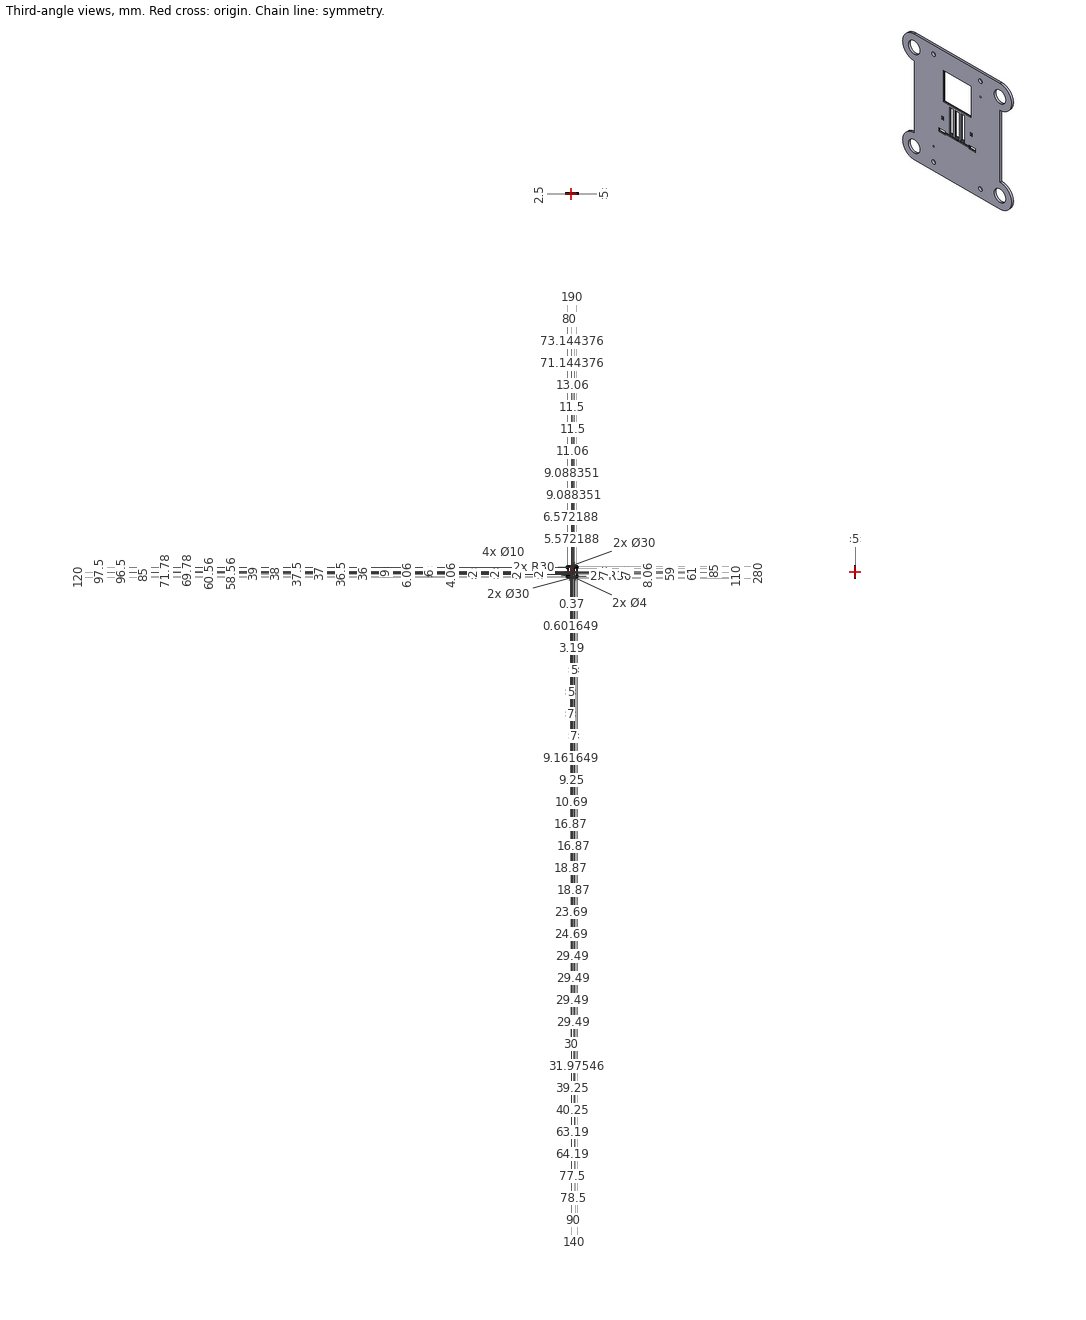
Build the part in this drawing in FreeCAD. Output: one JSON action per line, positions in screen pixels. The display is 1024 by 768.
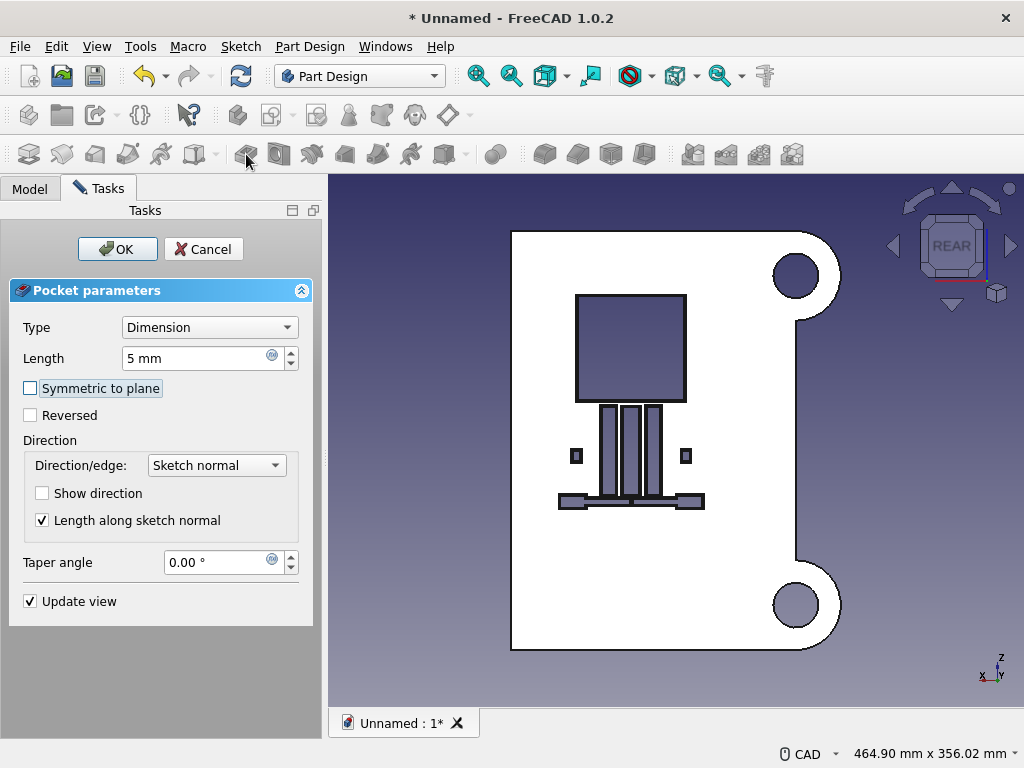
{"action": "left_click", "coordinate": [118, 249]}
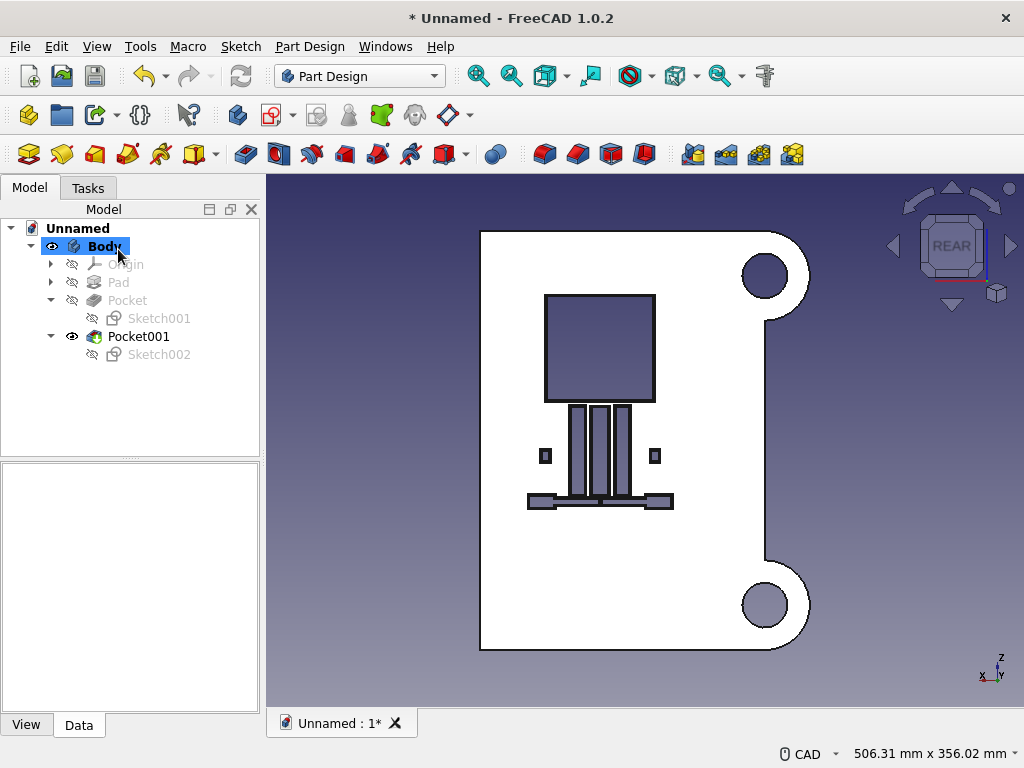
{"action": "left_click", "coordinate": [692, 559]}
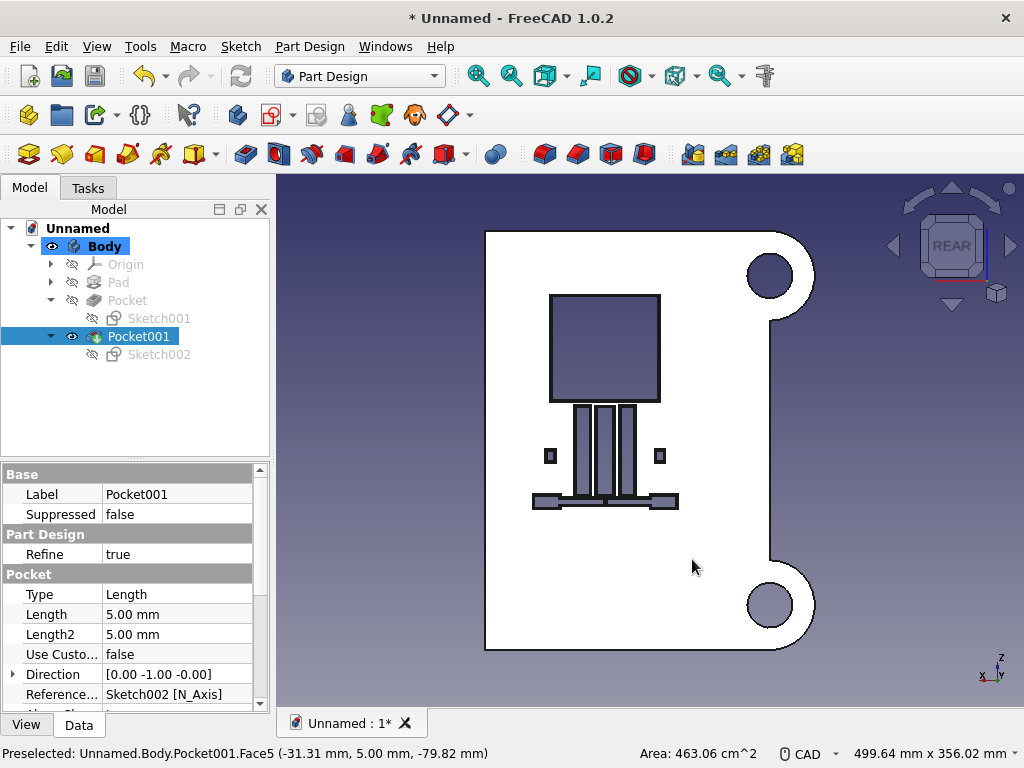
{"action": "left_click", "coordinate": [270, 116]}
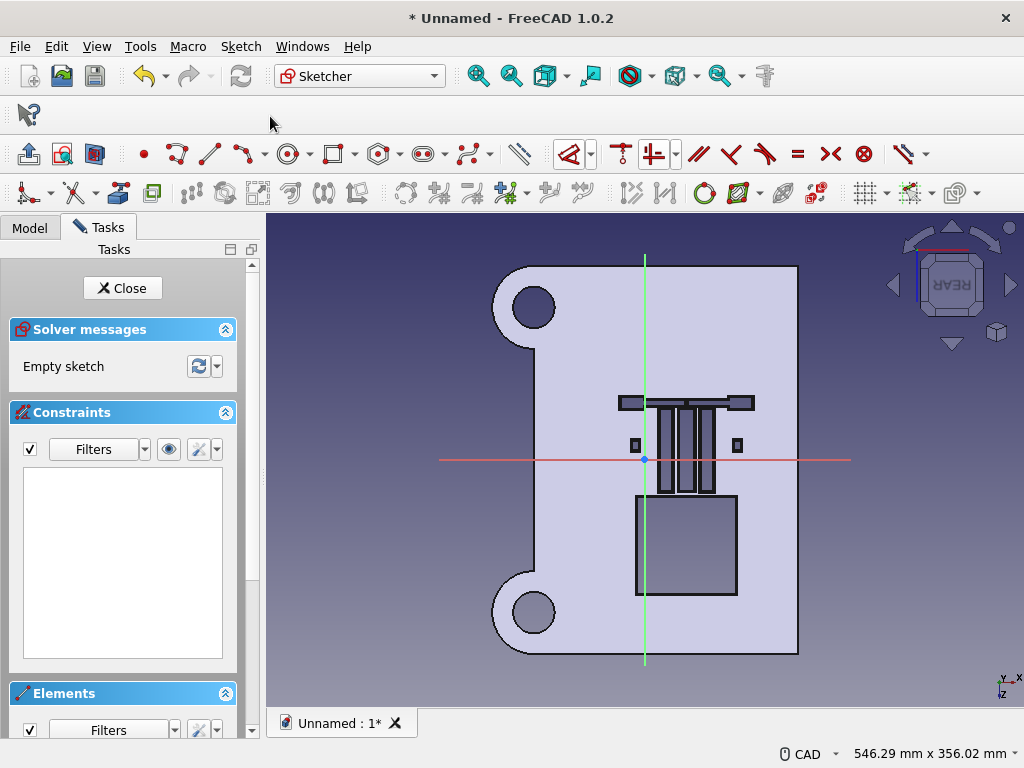
{"action": "key", "text": "g c"}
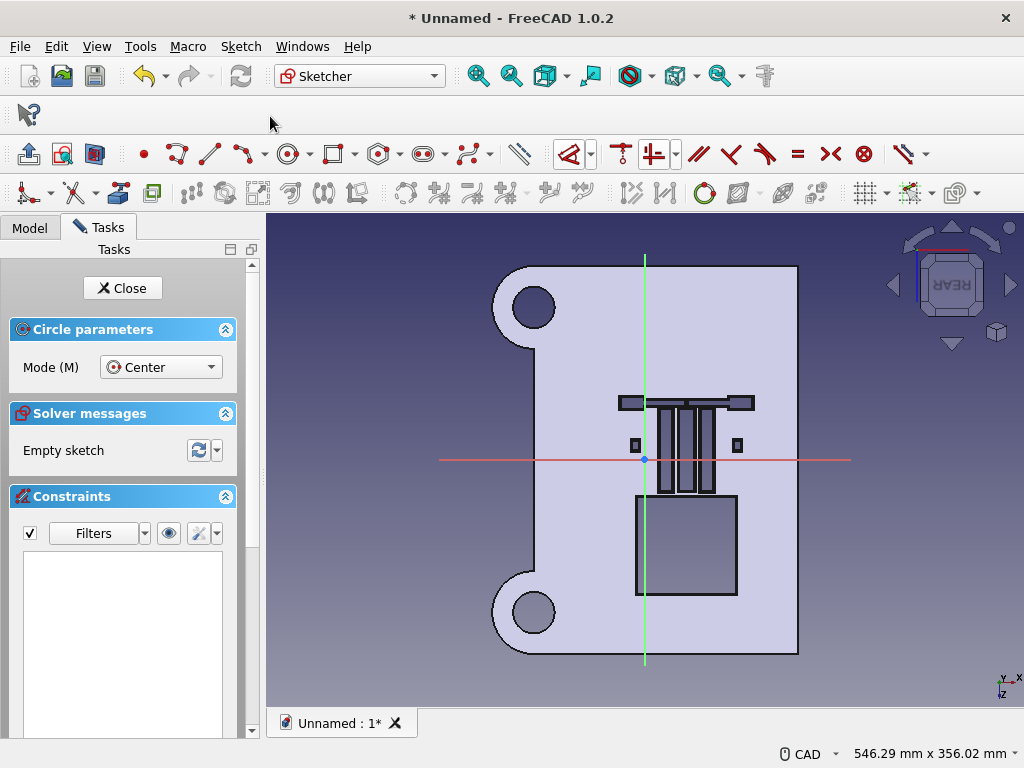
{"action": "scroll", "coordinate": [603, 293], "scroll_direction": "up", "scroll_amount": 6}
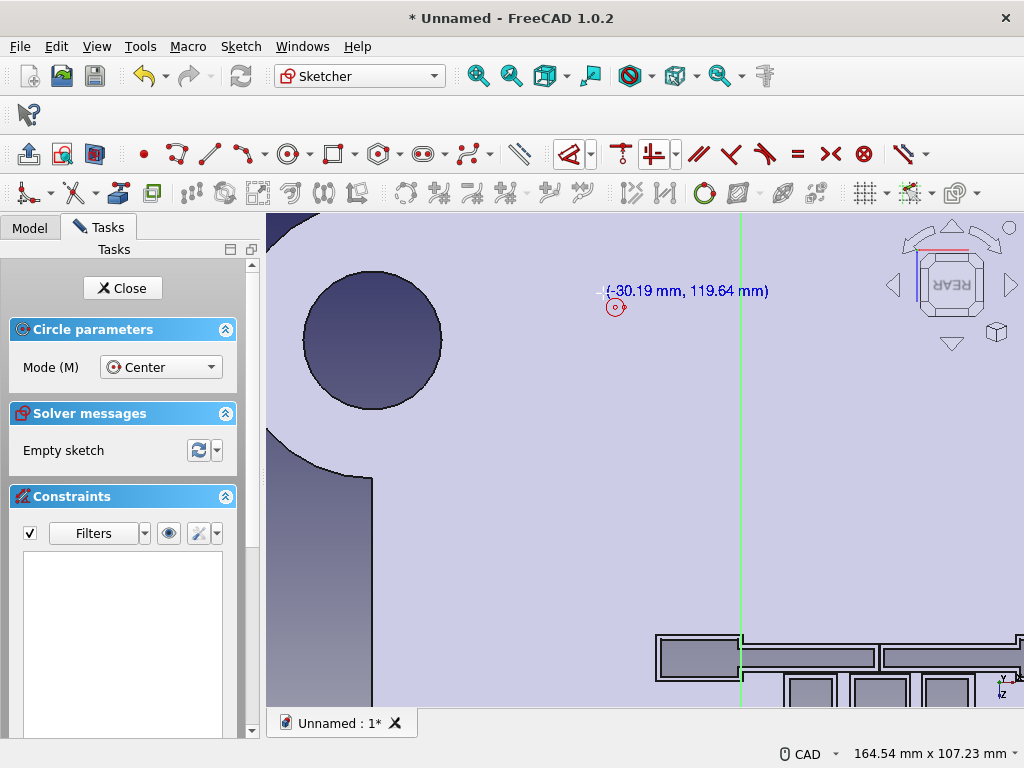
{"action": "left_click", "coordinate": [603, 294]}
{"action": "left_click", "coordinate": [619, 278]}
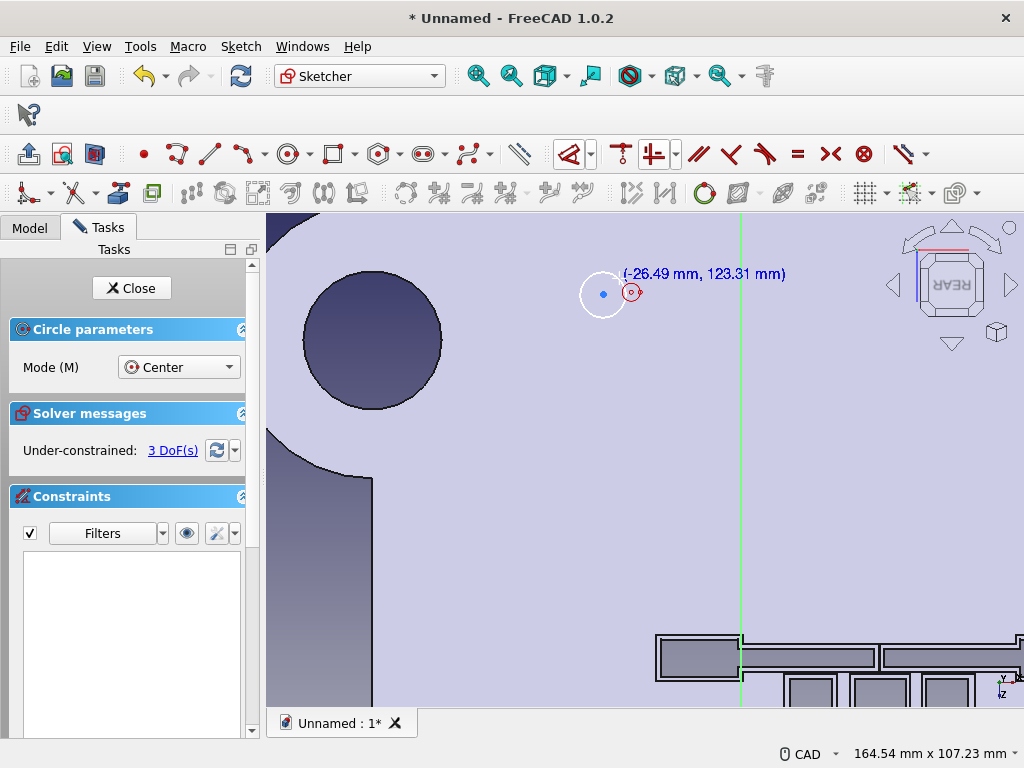
{"action": "scroll", "coordinate": [477, 333], "scroll_direction": "down", "scroll_amount": 7}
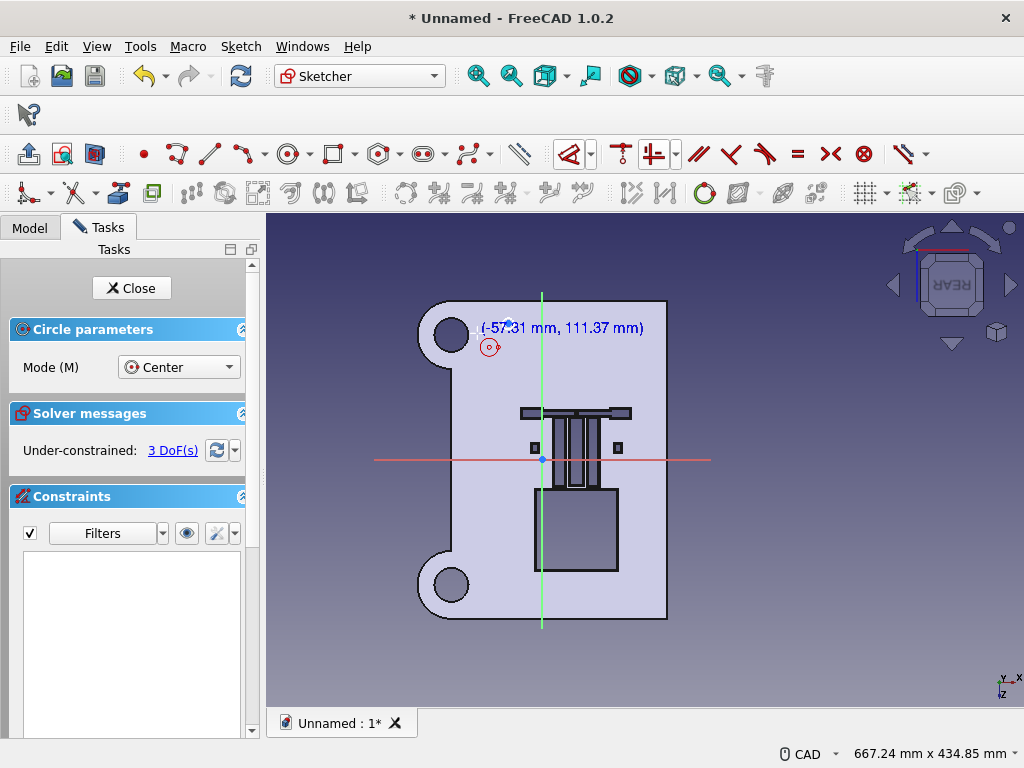
{"action": "scroll", "coordinate": [645, 324], "scroll_direction": "up", "scroll_amount": 7}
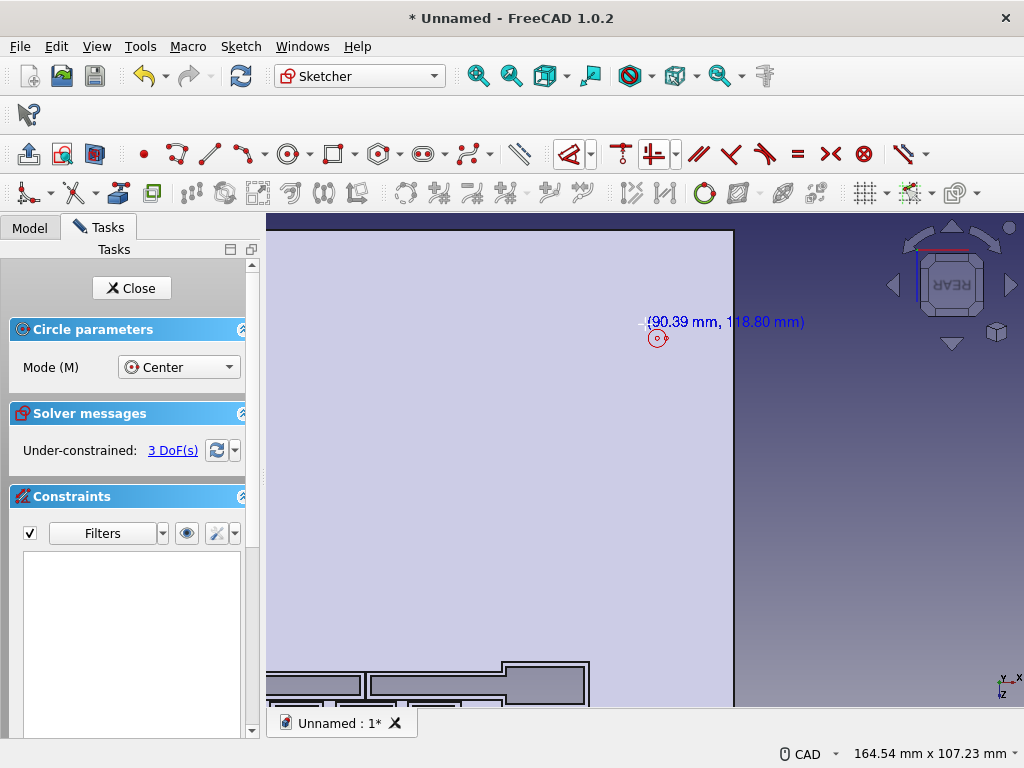
{"action": "left_click", "coordinate": [642, 322]}
{"action": "left_click", "coordinate": [658, 306]}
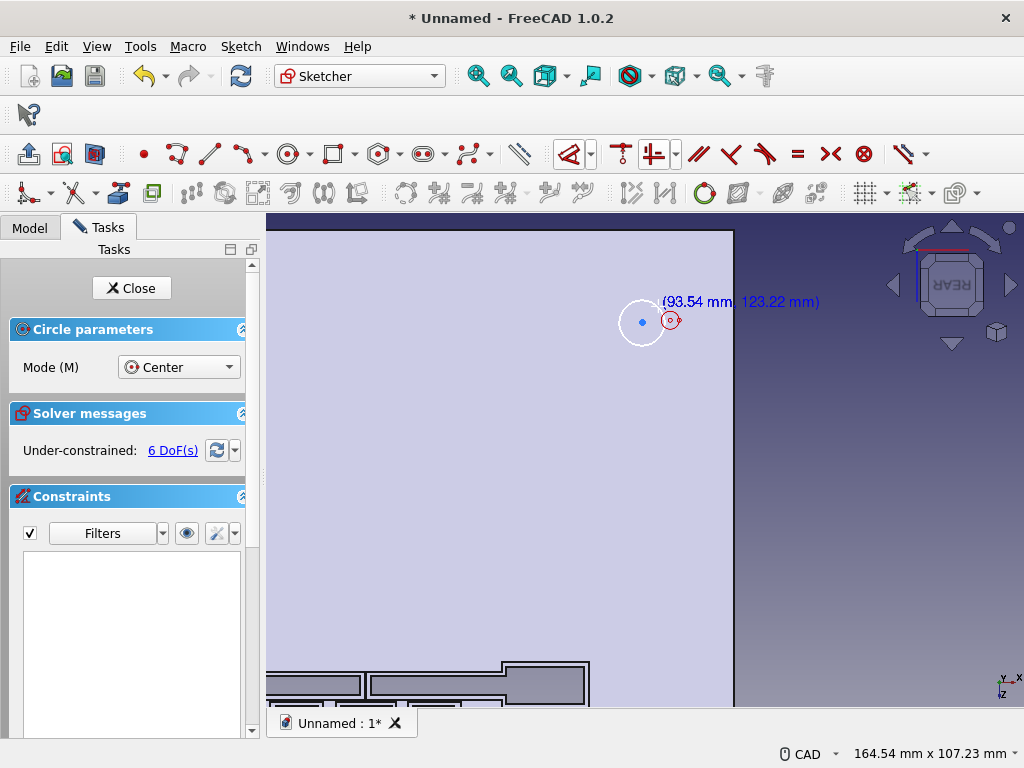
{"action": "scroll", "coordinate": [646, 324], "scroll_direction": "down", "scroll_amount": 7}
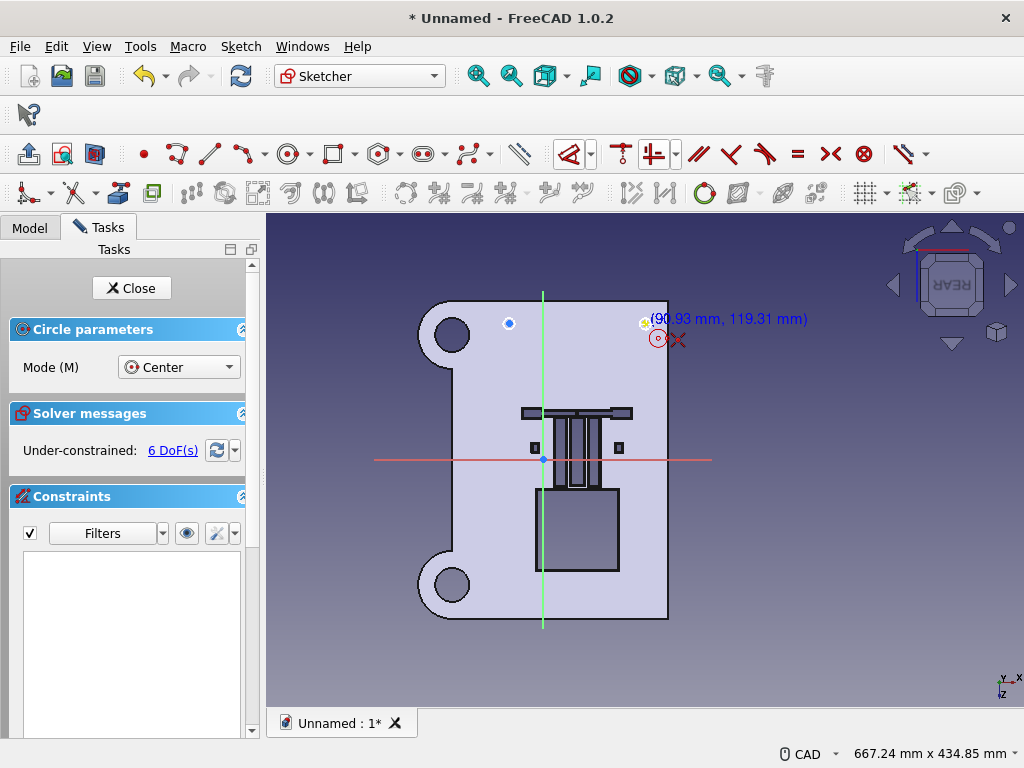
{"action": "scroll", "coordinate": [645, 596], "scroll_direction": "up", "scroll_amount": 7}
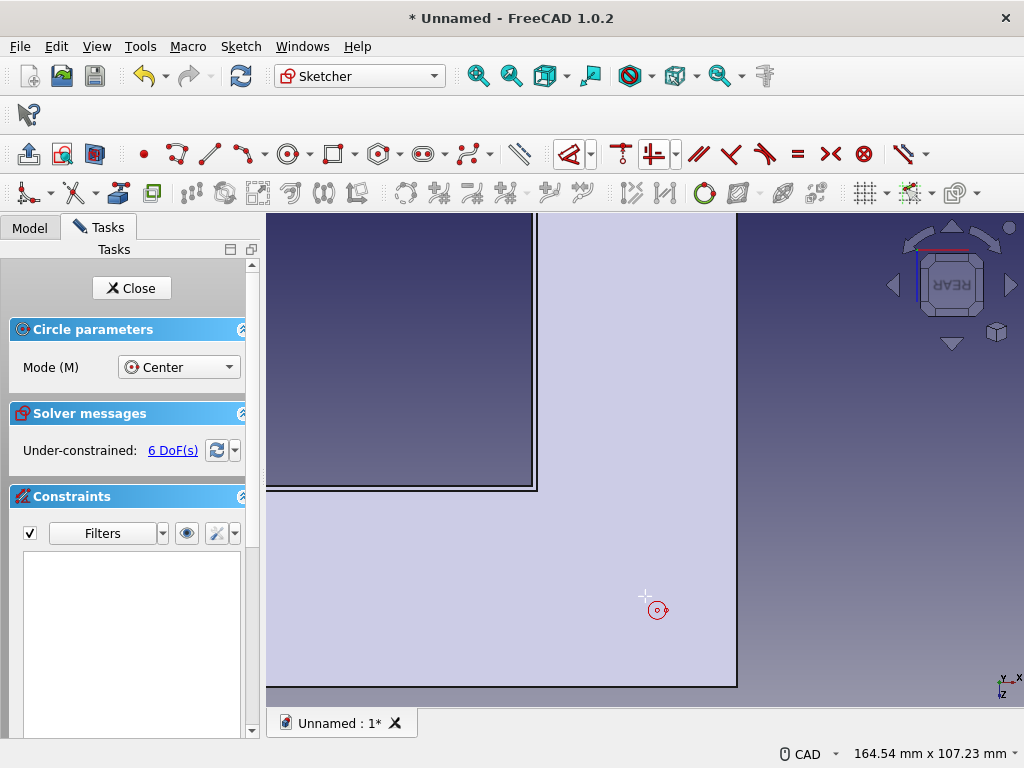
{"action": "left_click", "coordinate": [645, 595]}
{"action": "left_click", "coordinate": [661, 578]}